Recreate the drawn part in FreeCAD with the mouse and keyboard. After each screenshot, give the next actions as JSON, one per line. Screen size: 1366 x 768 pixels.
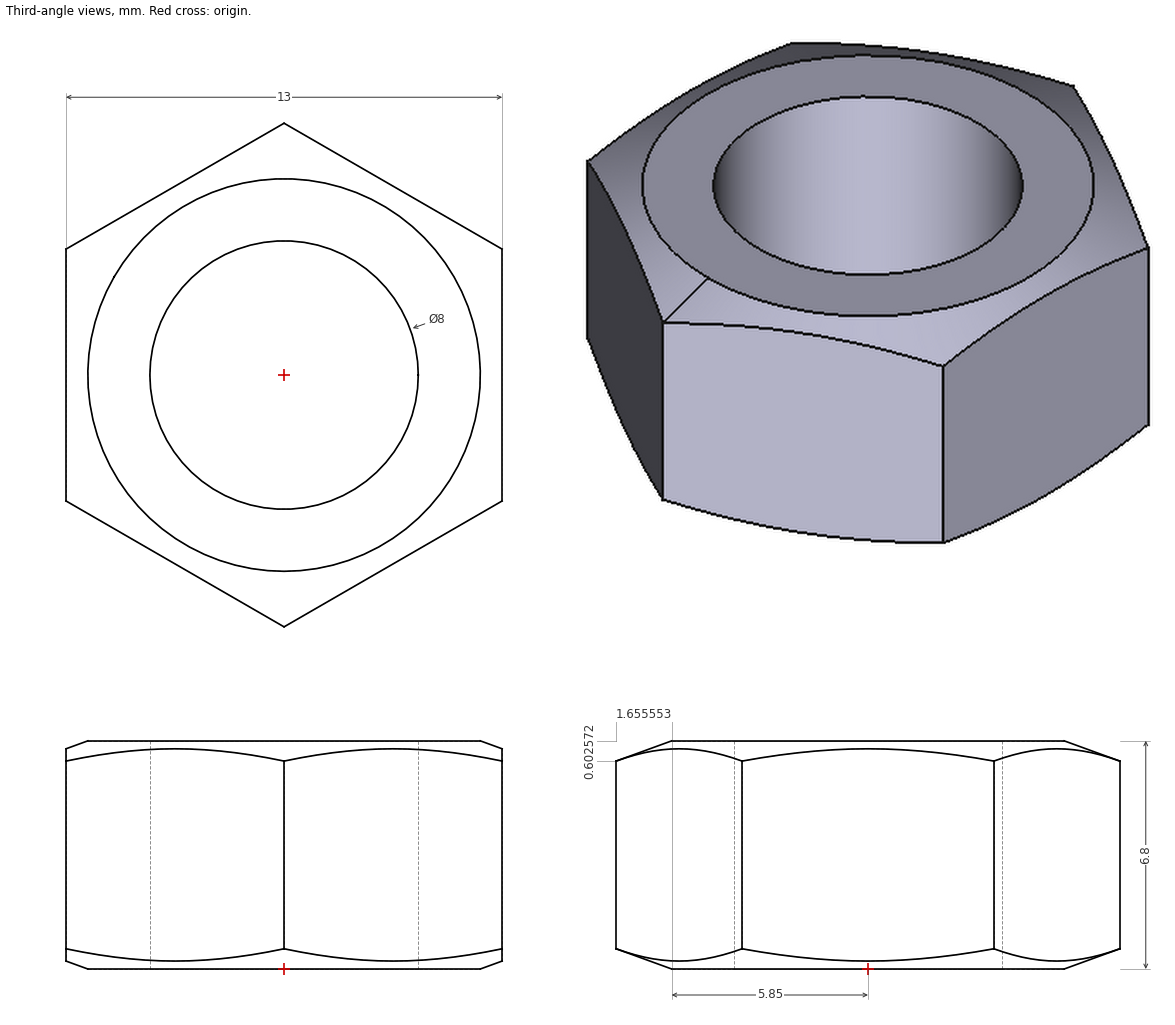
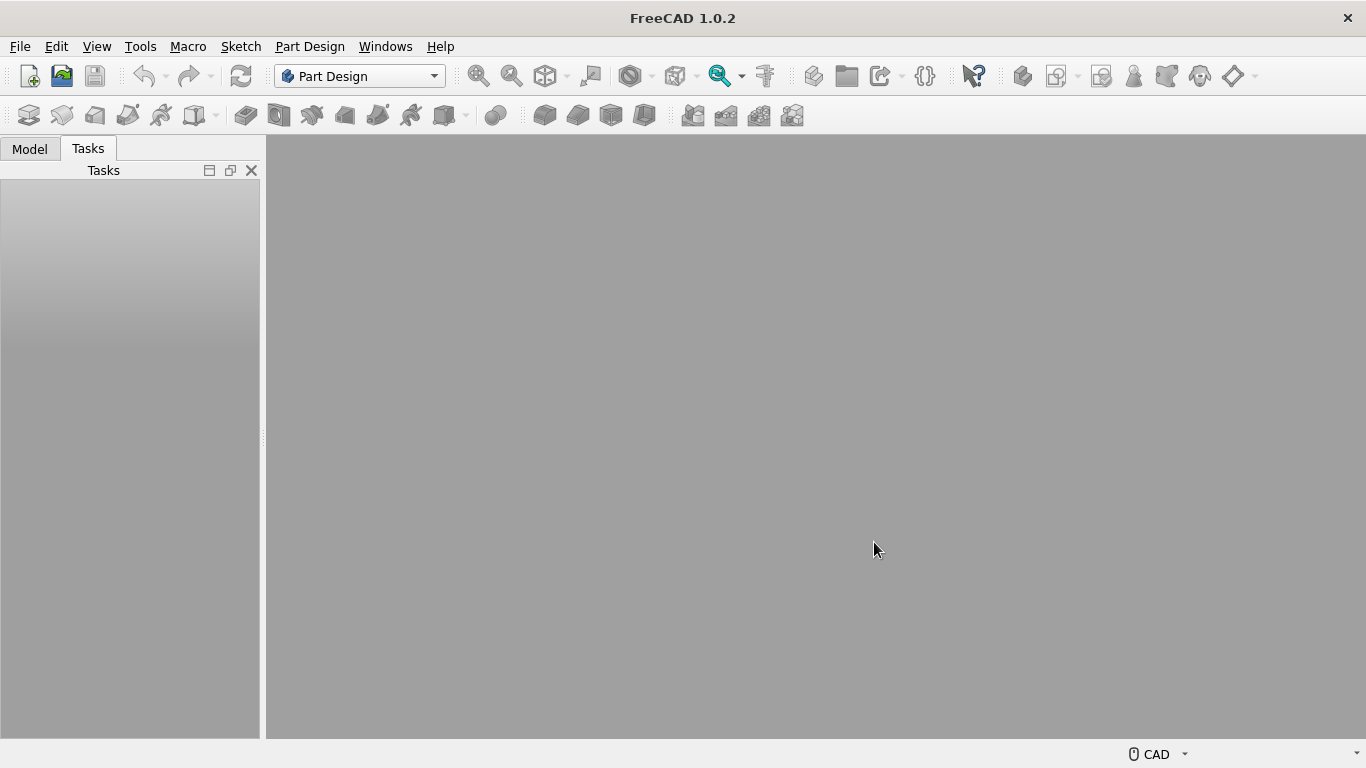
{"action": "left_click", "coordinate": [29, 76]}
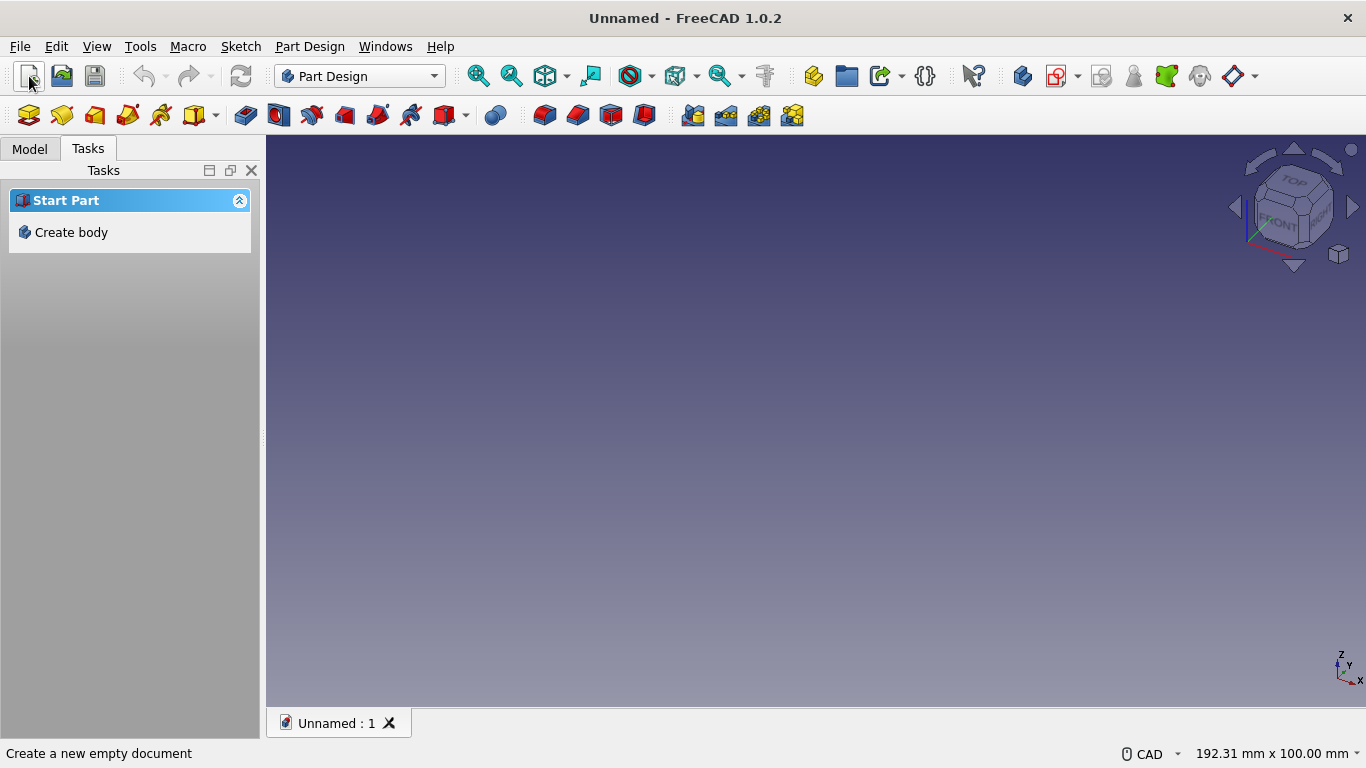
{"action": "left_click", "coordinate": [1056, 76]}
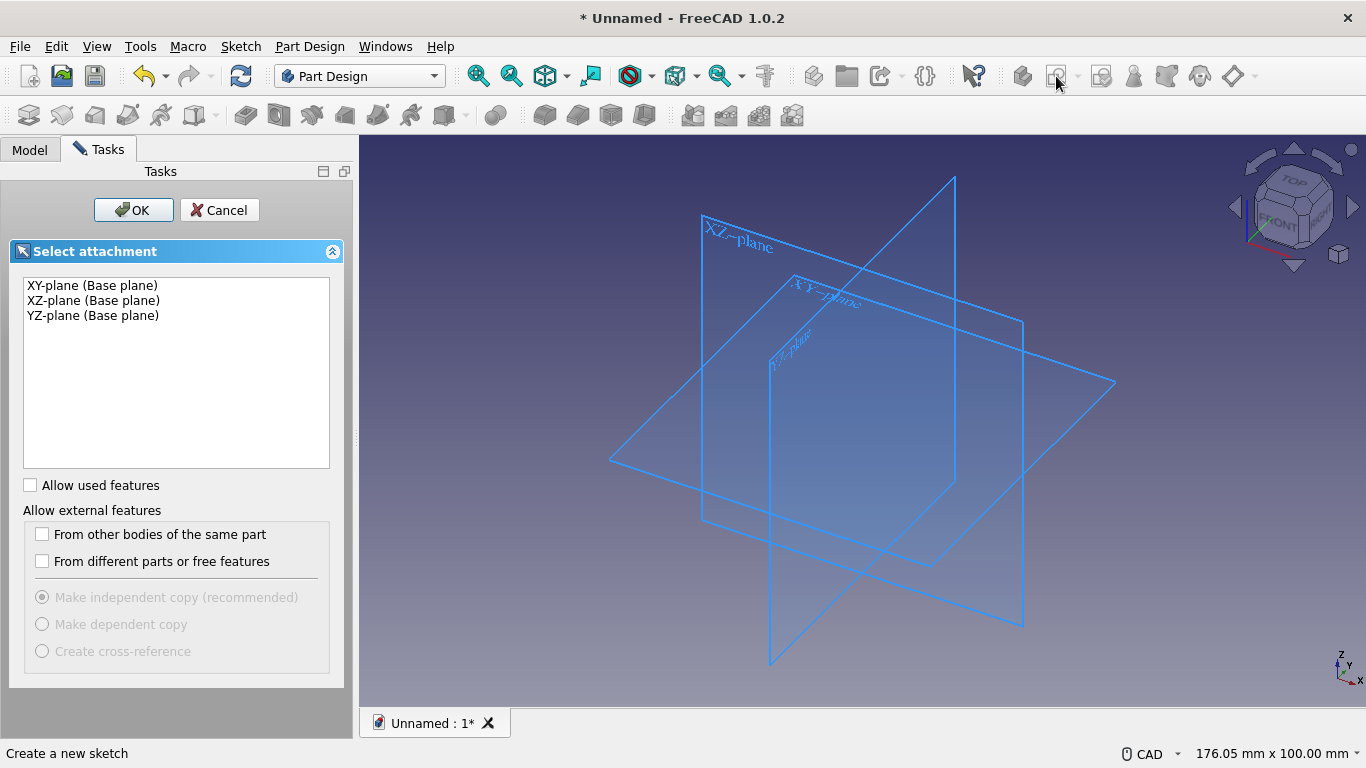
{"action": "left_click", "coordinate": [84, 286]}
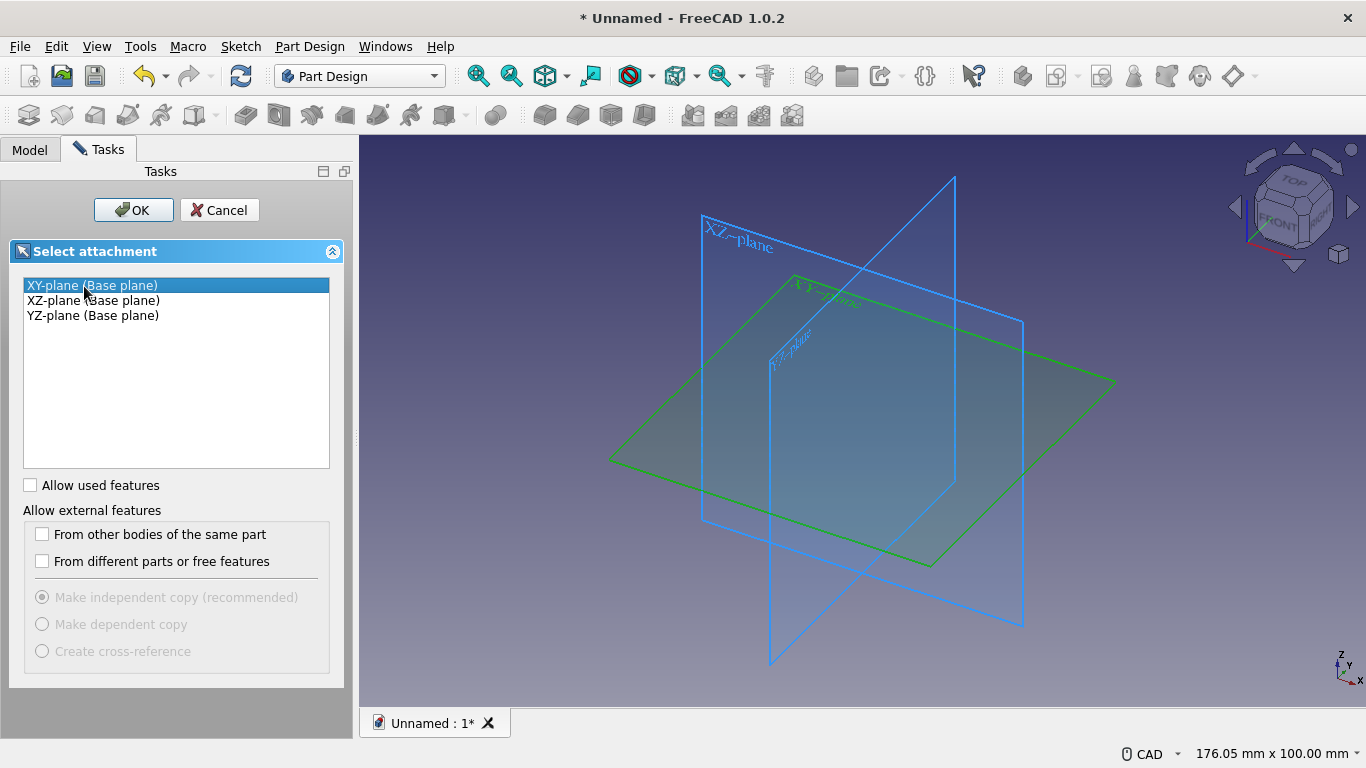
{"action": "left_click", "coordinate": [134, 210]}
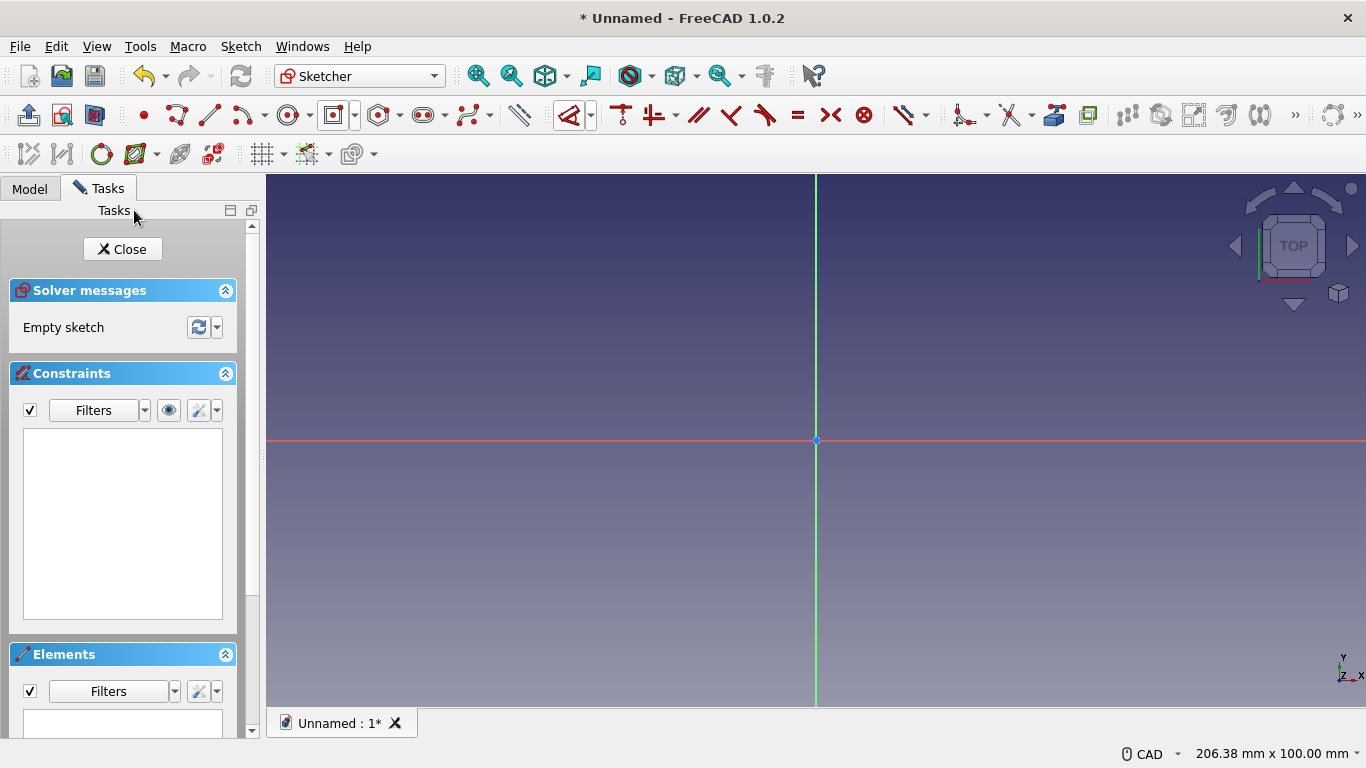
{"action": "scroll", "coordinate": [838, 440], "scroll_direction": "up", "scroll_amount": 7}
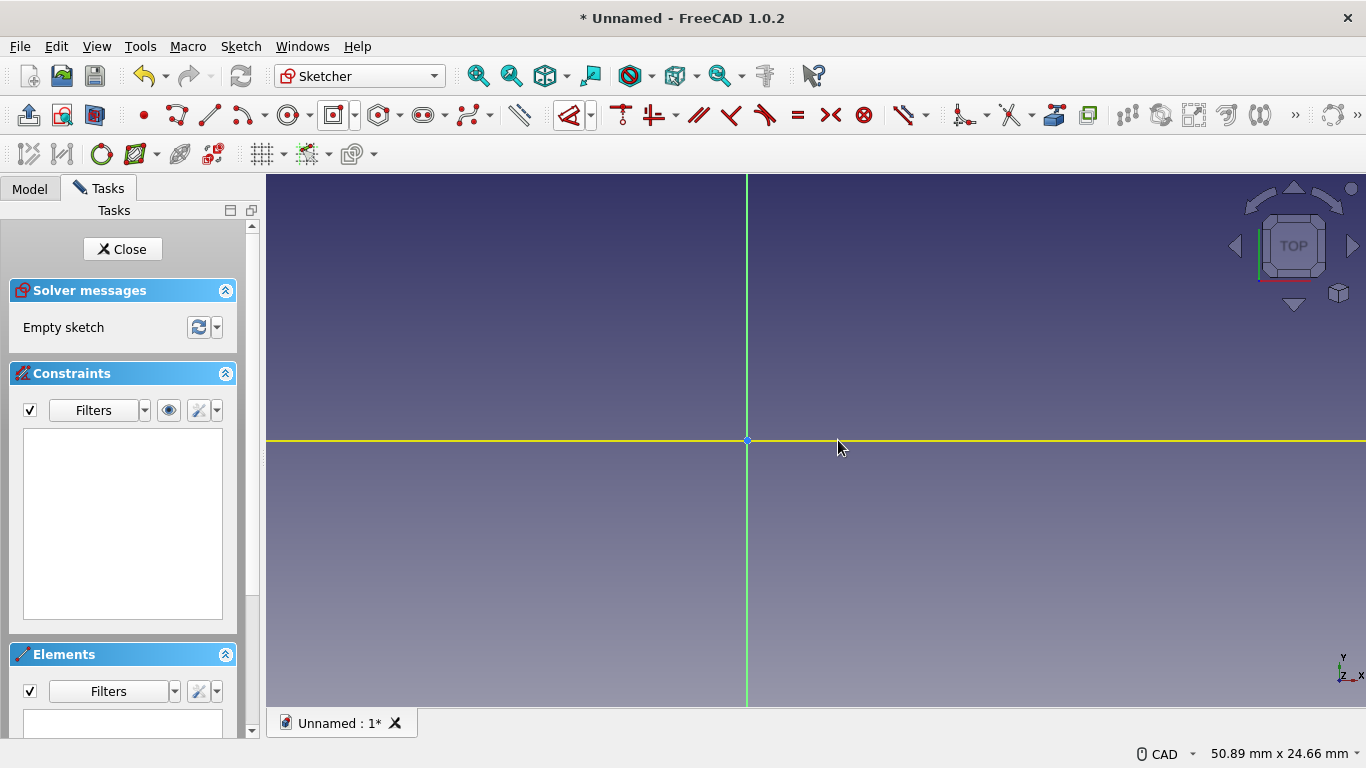
{"action": "key", "text": "g p 6"}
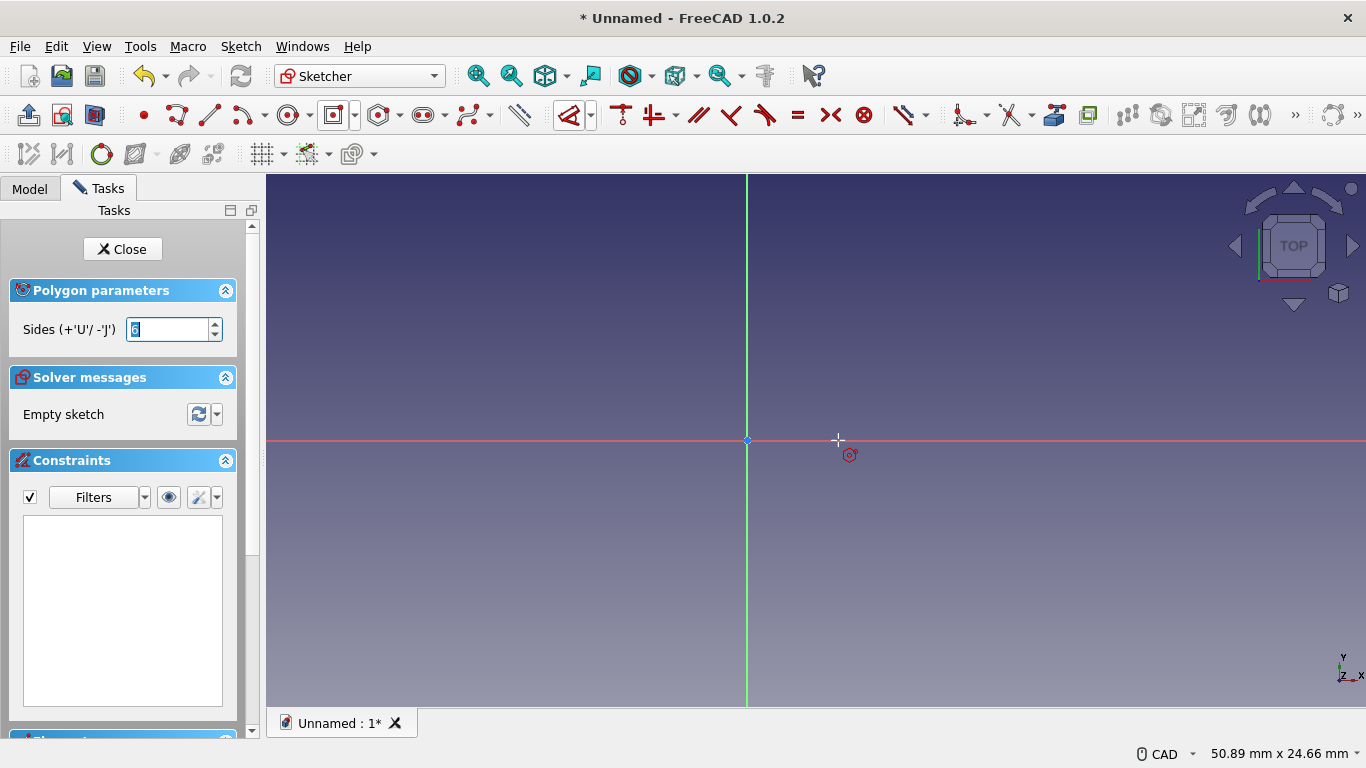
{"action": "left_click", "coordinate": [747, 440]}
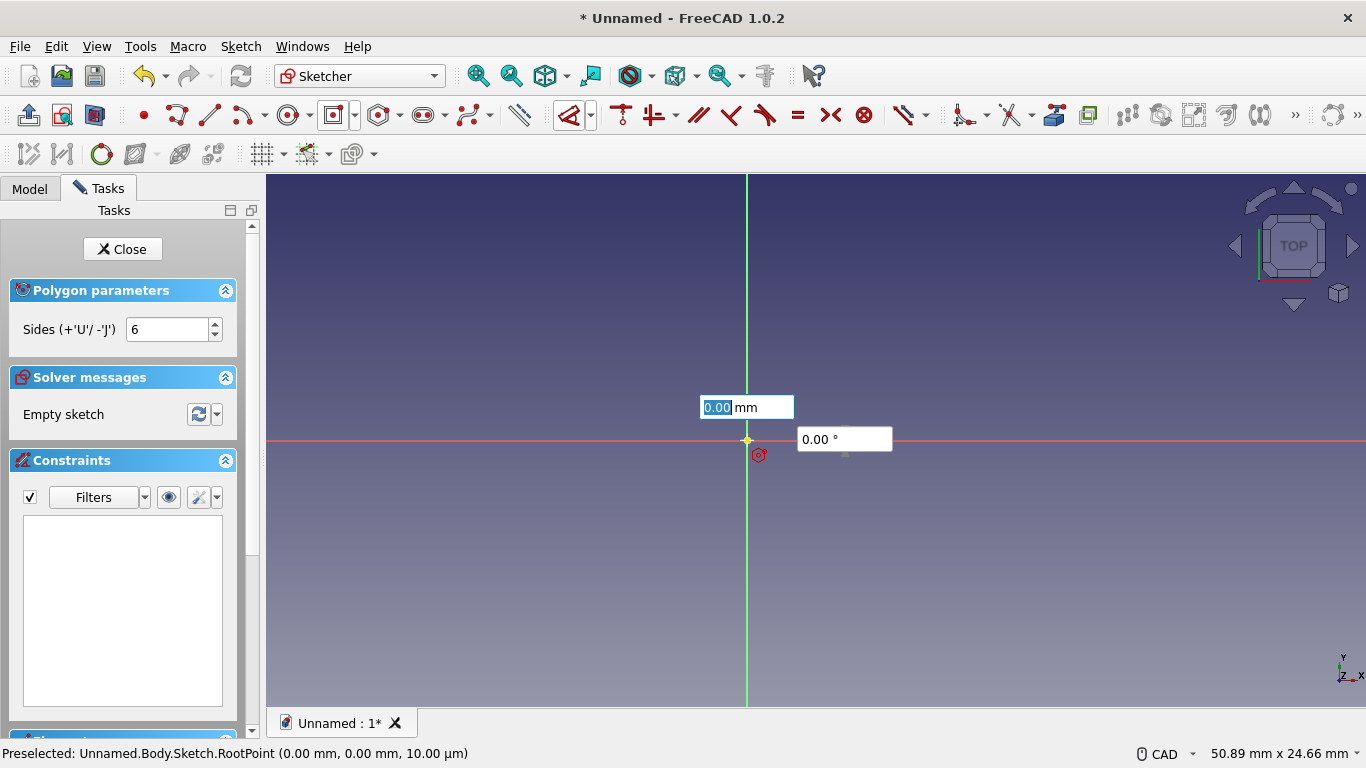
{"action": "left_click", "coordinate": [747, 278]}
{"action": "right_click", "coordinate": [747, 278]}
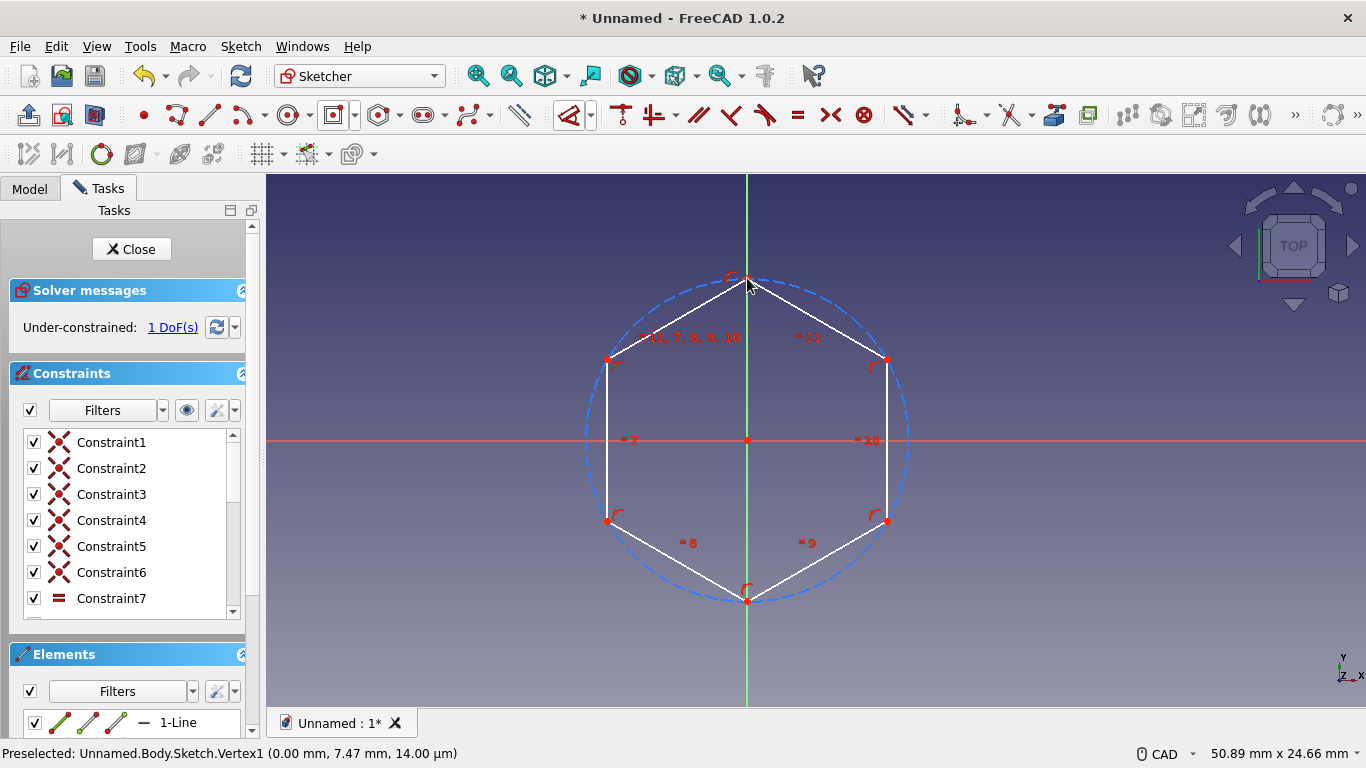
{"action": "left_click", "coordinate": [568, 116]}